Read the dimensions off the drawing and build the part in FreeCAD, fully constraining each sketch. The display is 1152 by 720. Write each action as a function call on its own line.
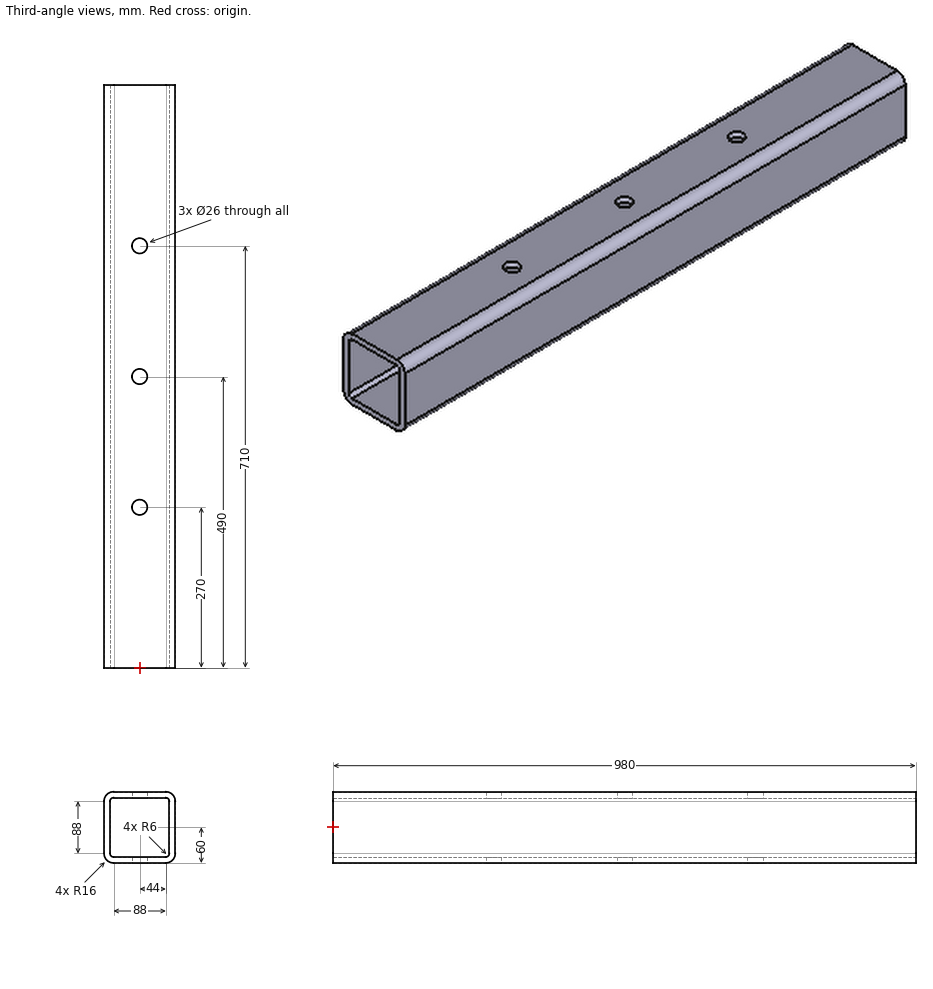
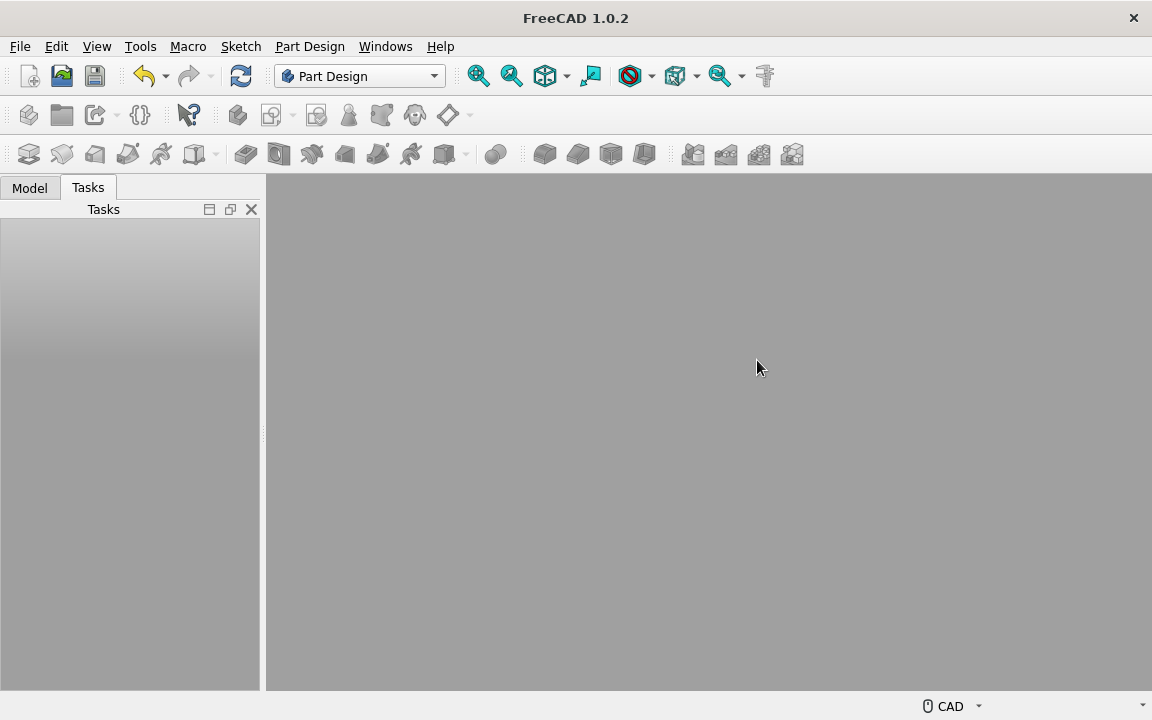
click(29, 76)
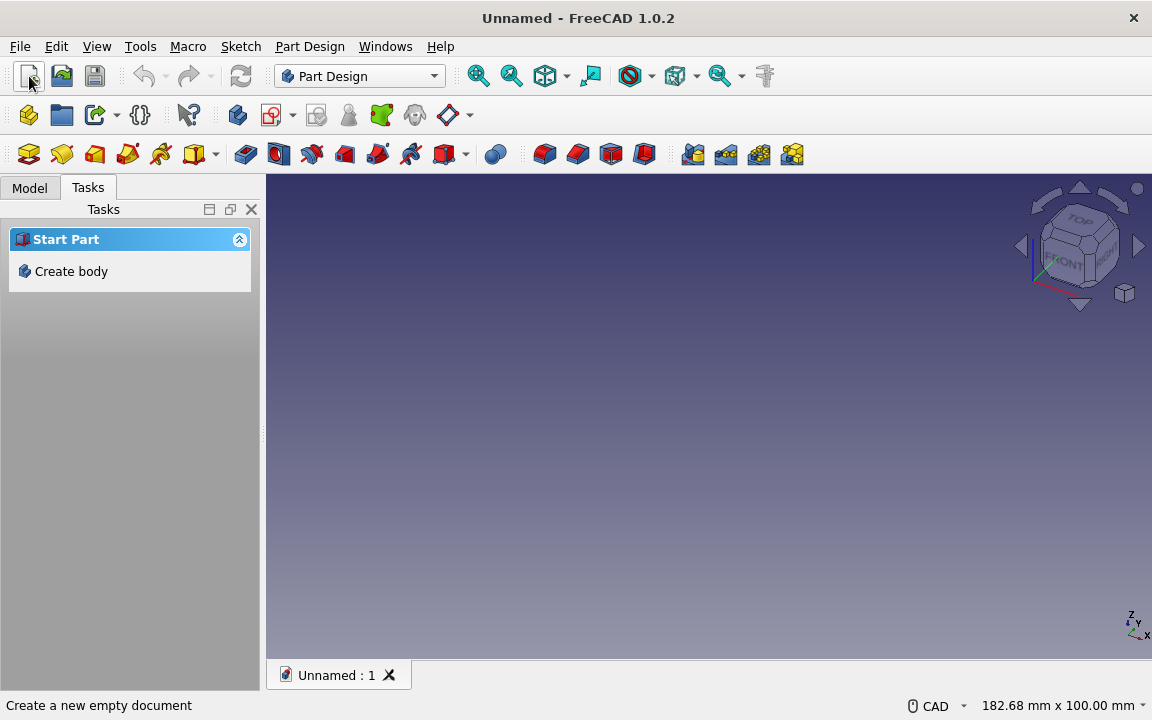
click(270, 116)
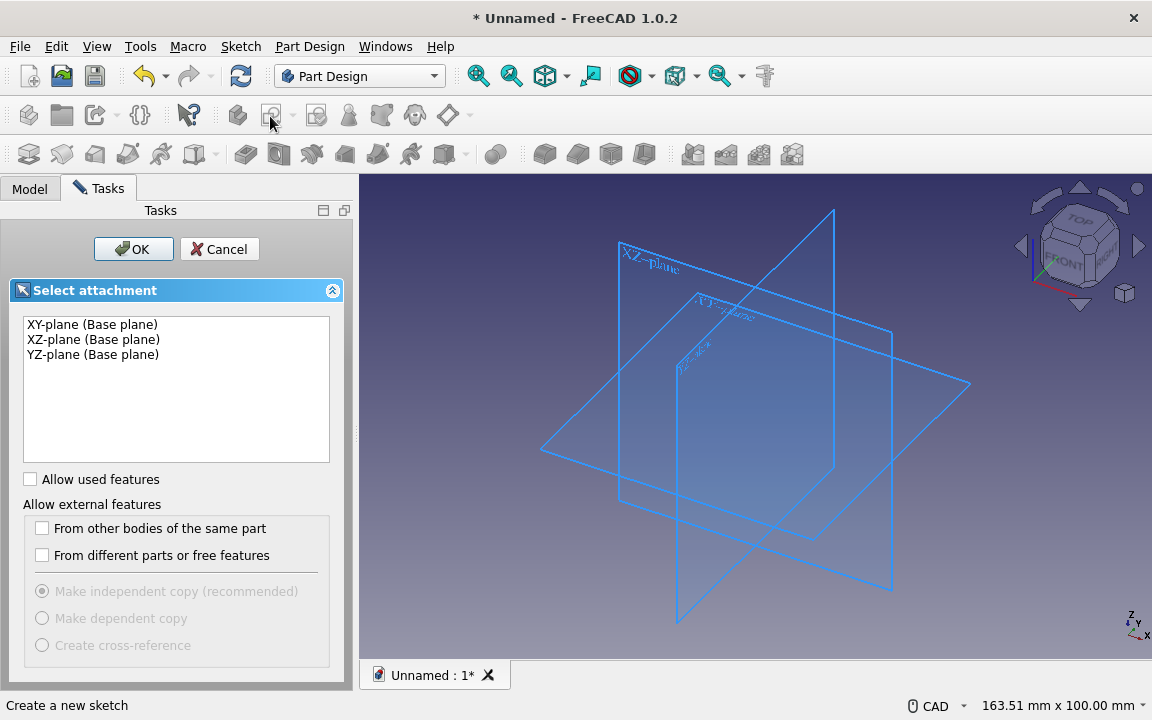
click(84, 340)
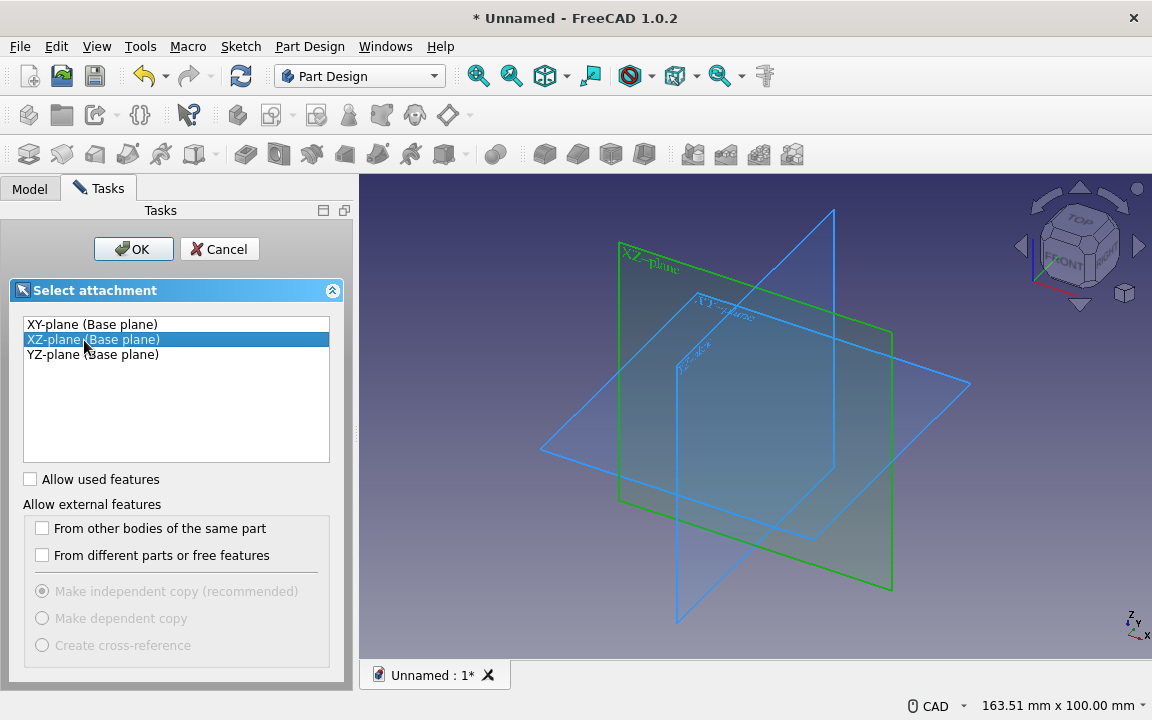
click(134, 249)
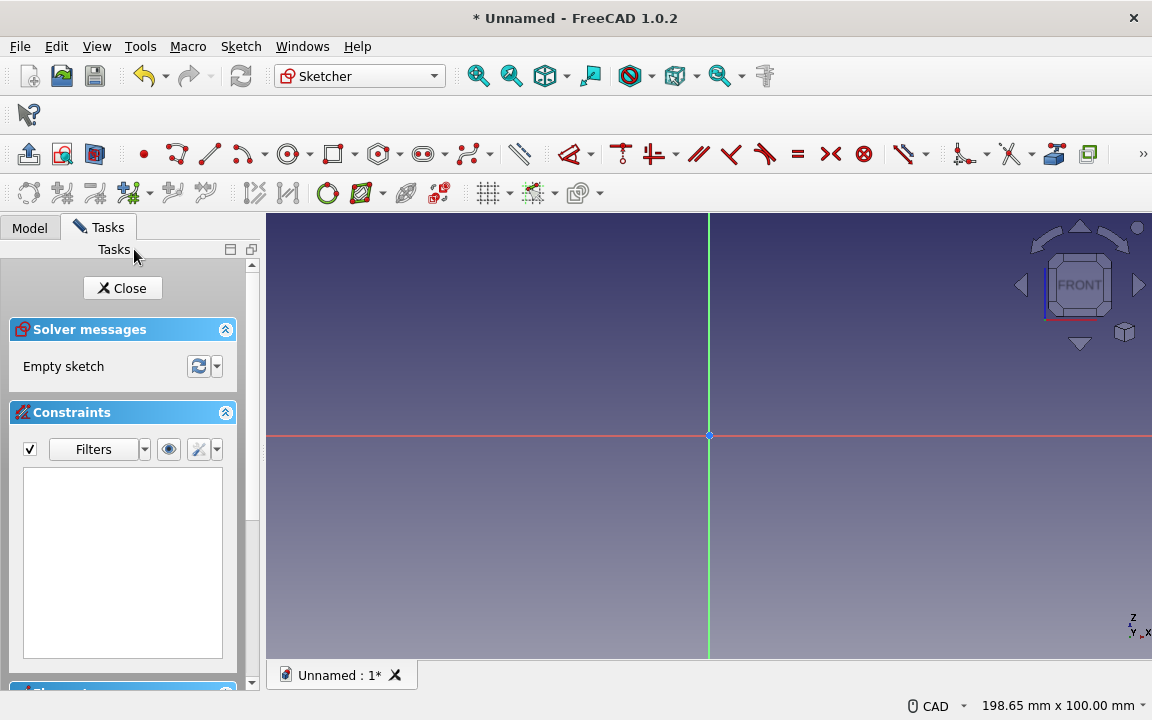
scroll(557, 436, down, 3)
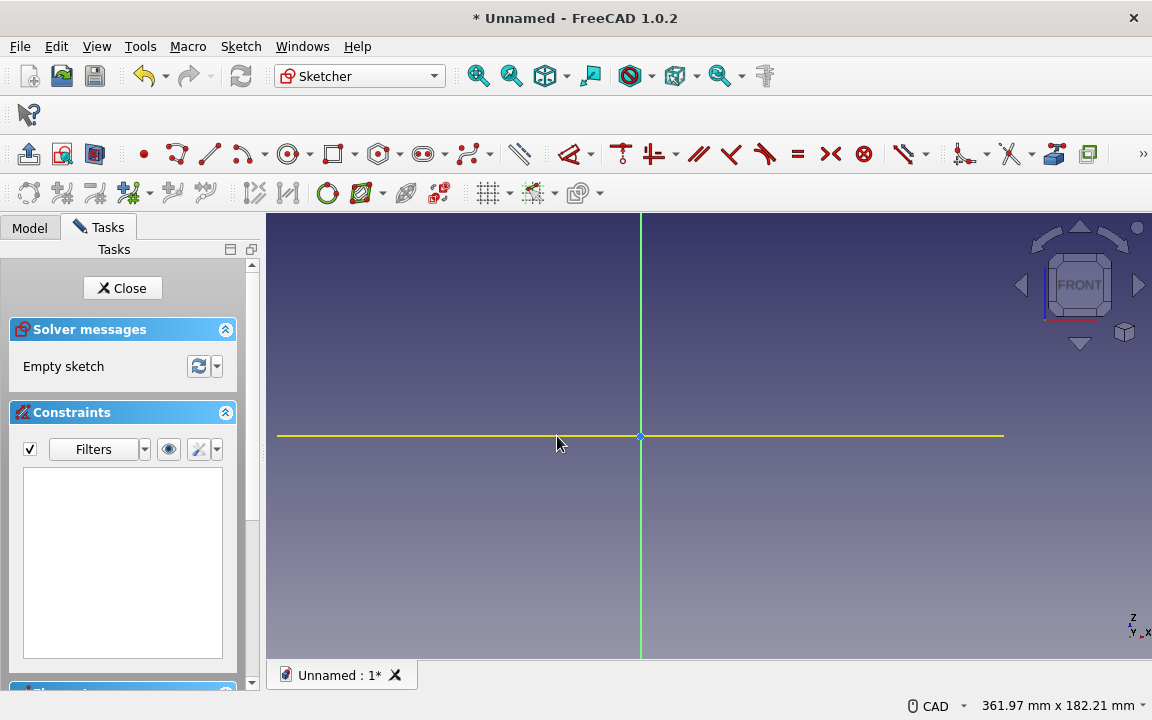
click(210, 154)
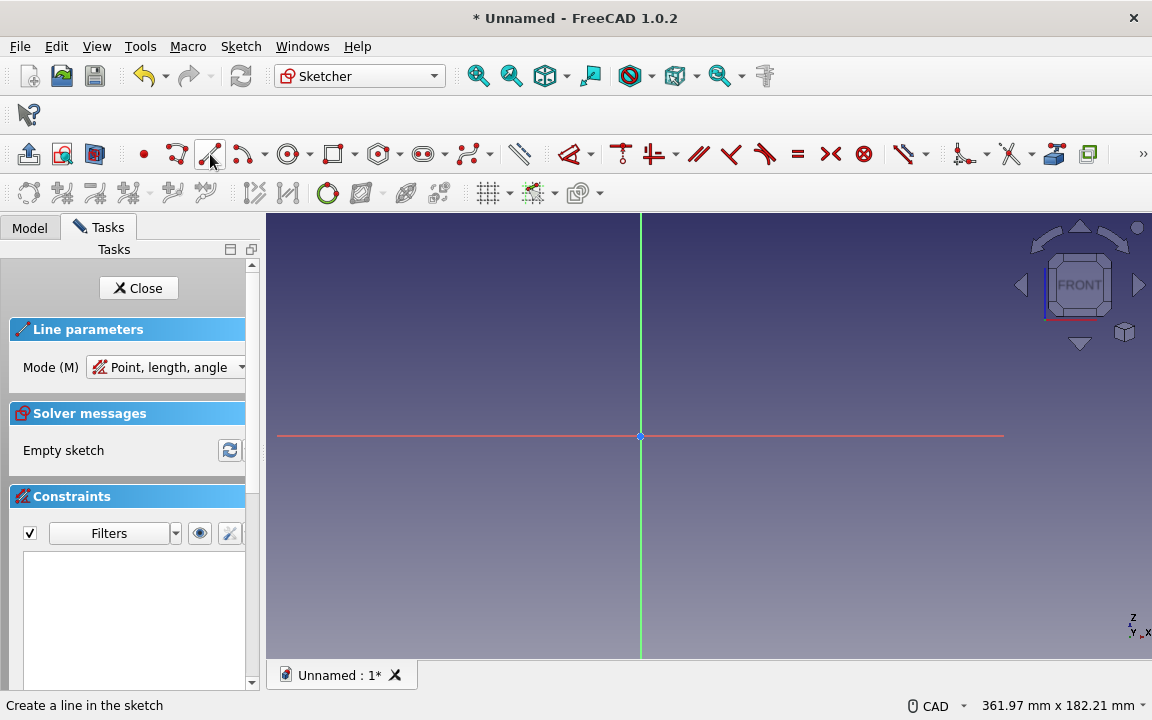
click(748, 583)
click(533, 583)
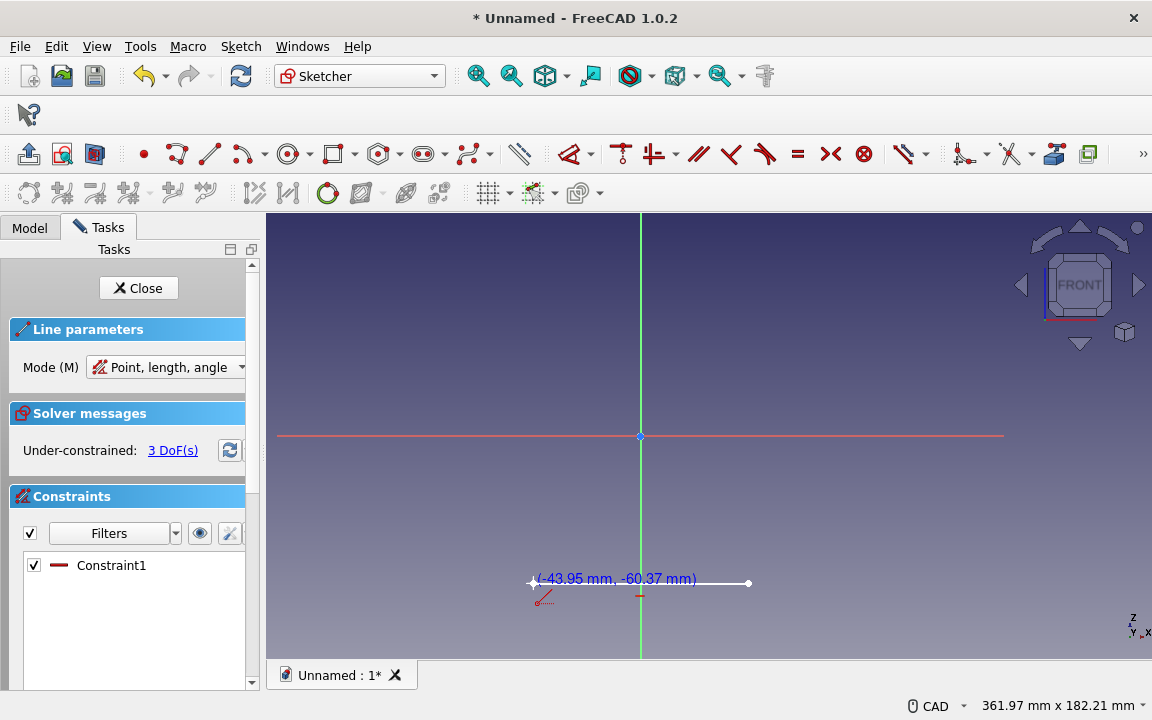
click(494, 544)
click(494, 329)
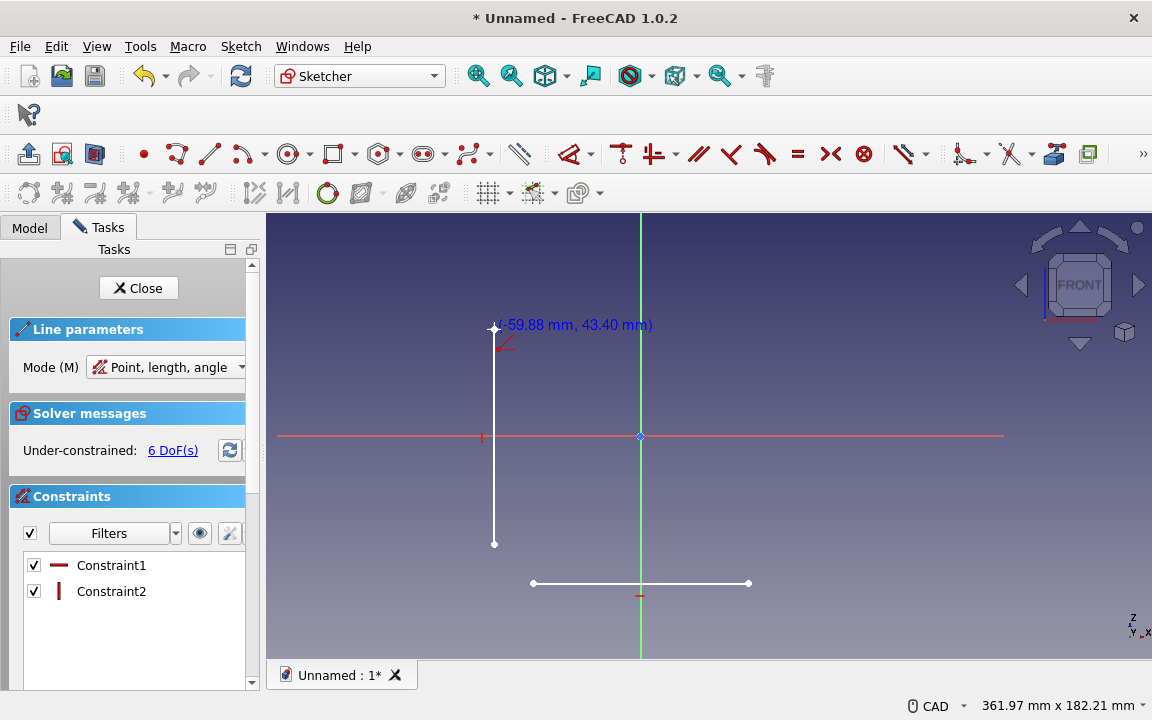
click(533, 289)
click(748, 289)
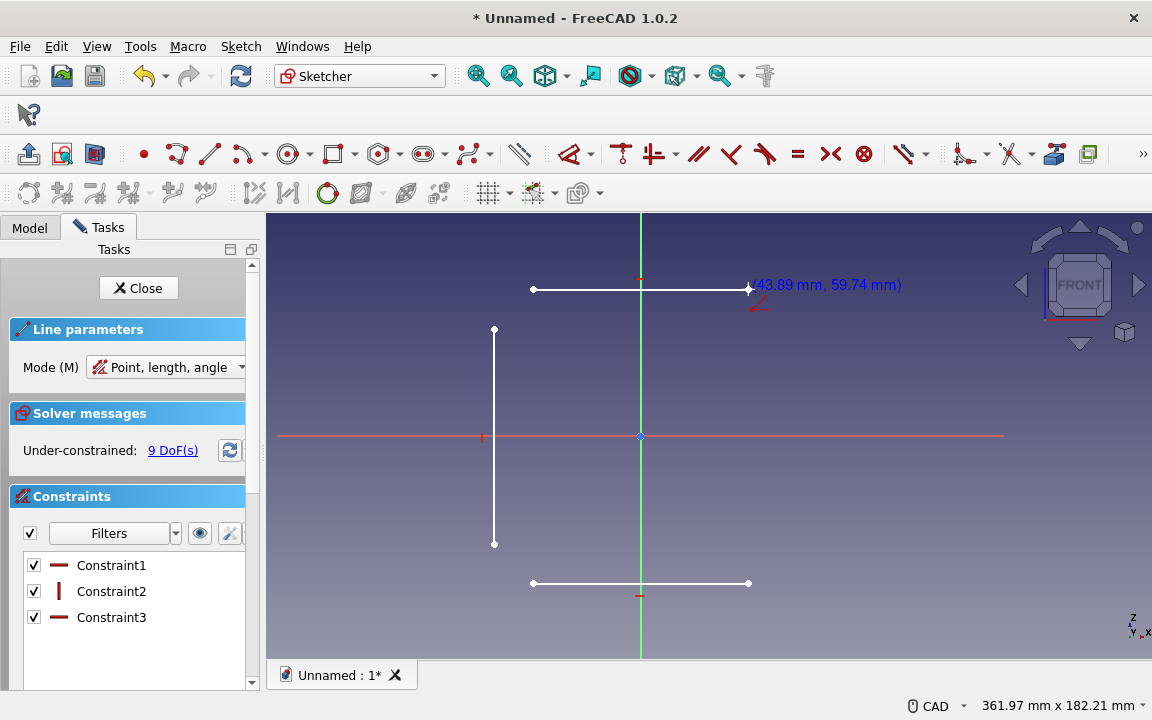
click(787, 329)
click(787, 544)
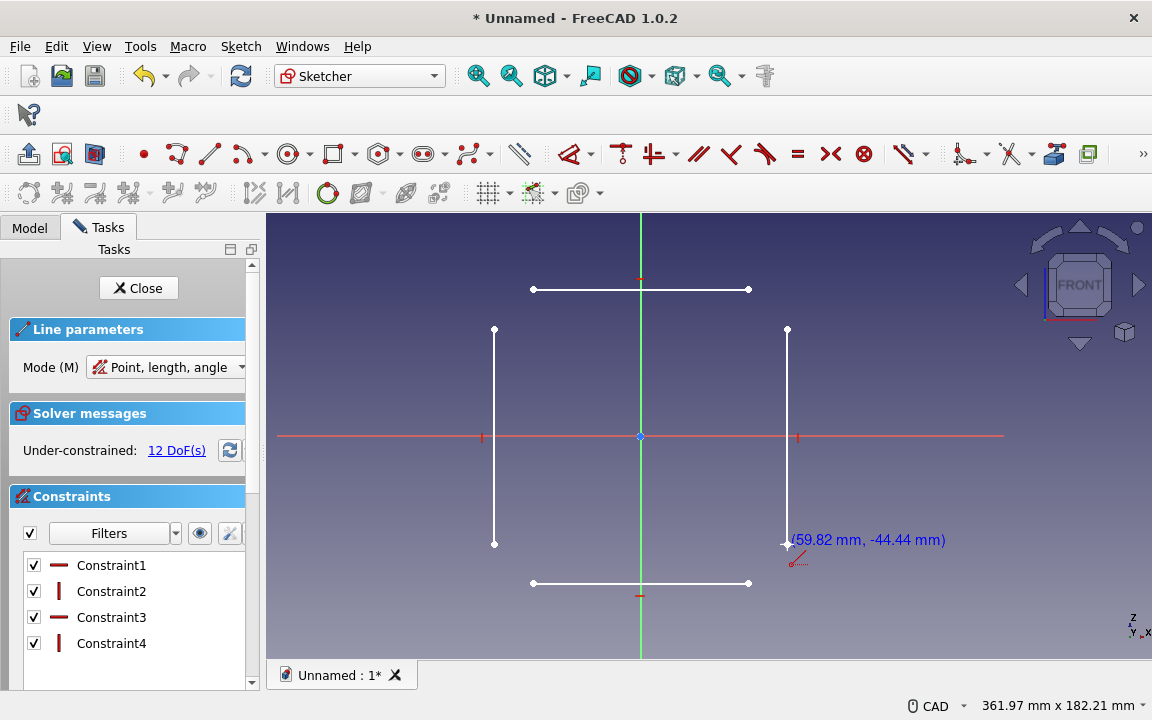
key(g)
key(3)
key(a)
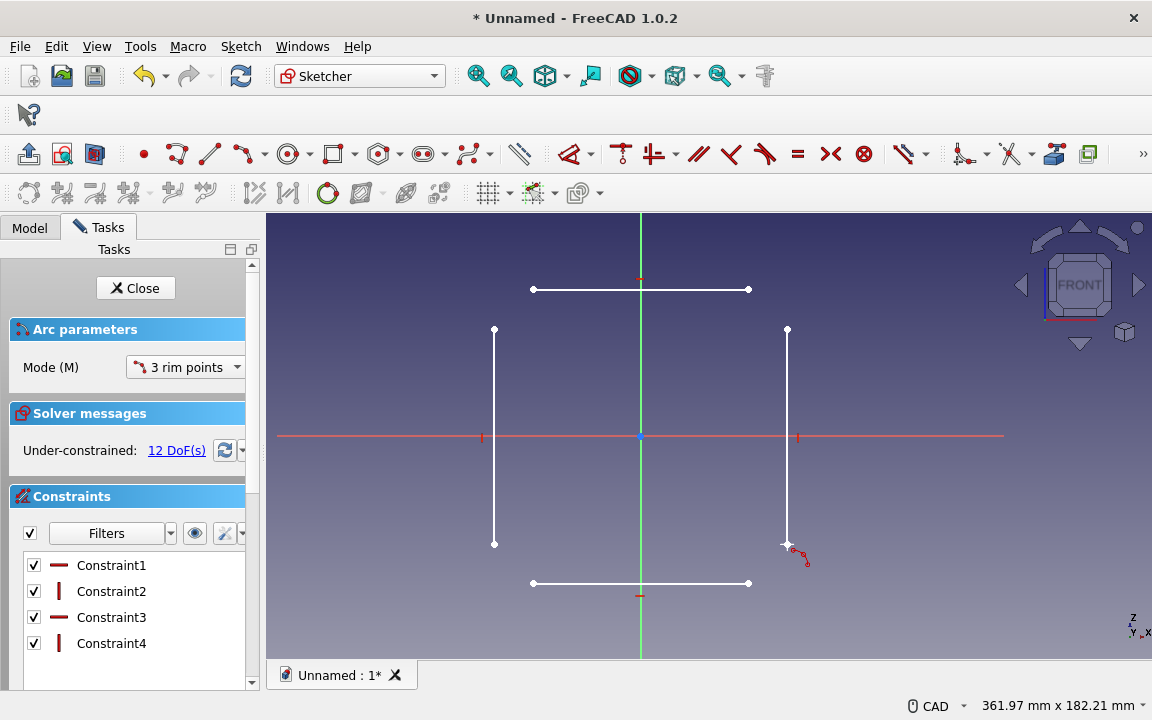
click(533, 584)
click(494, 545)